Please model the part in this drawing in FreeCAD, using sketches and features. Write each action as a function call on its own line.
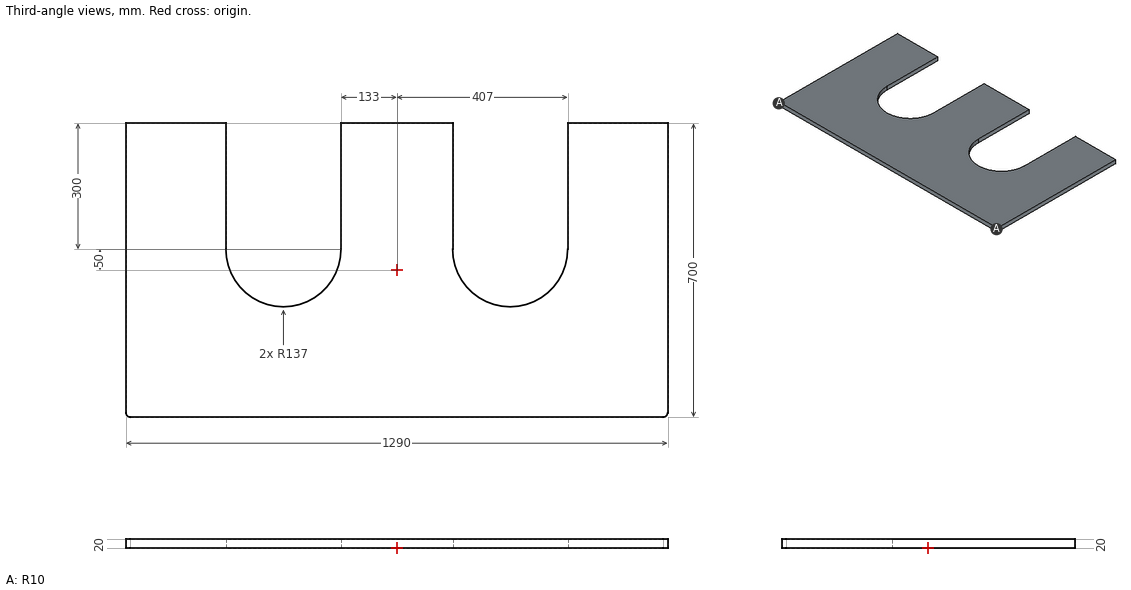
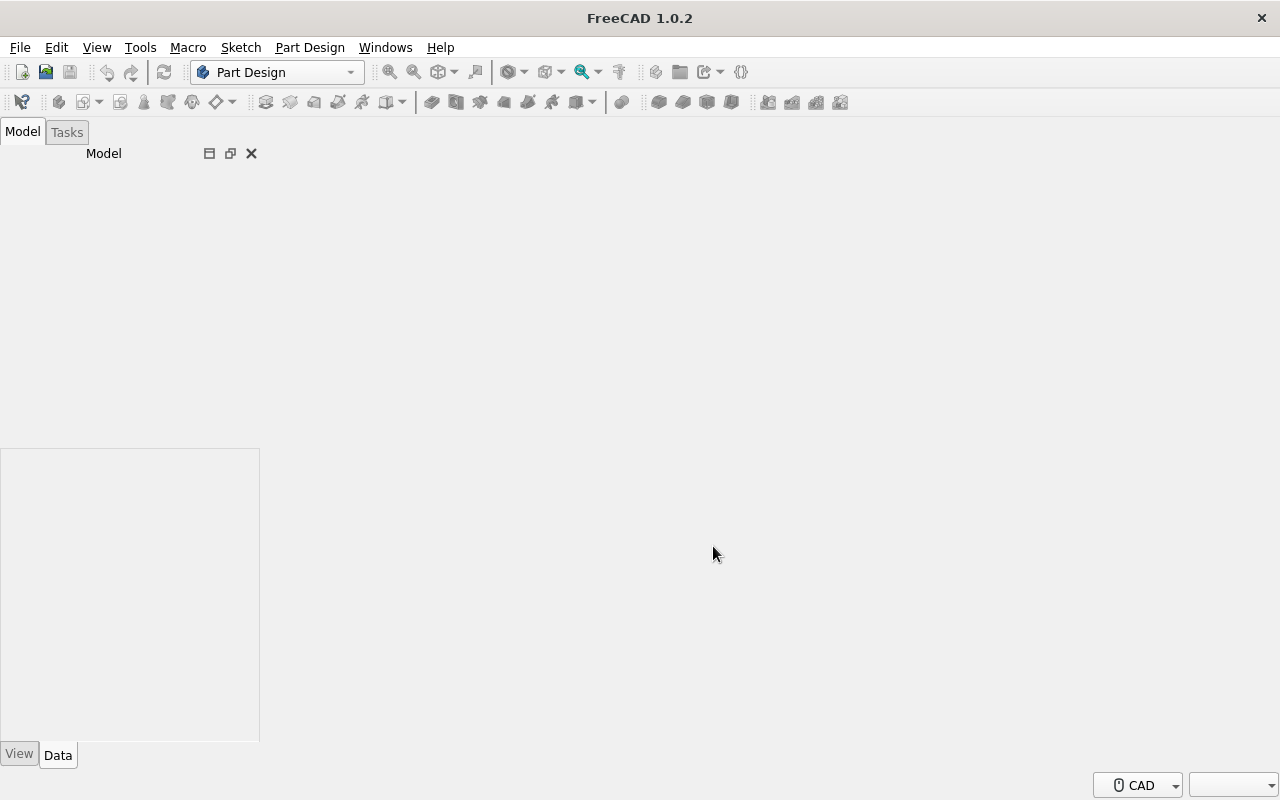
key(ctrl+n)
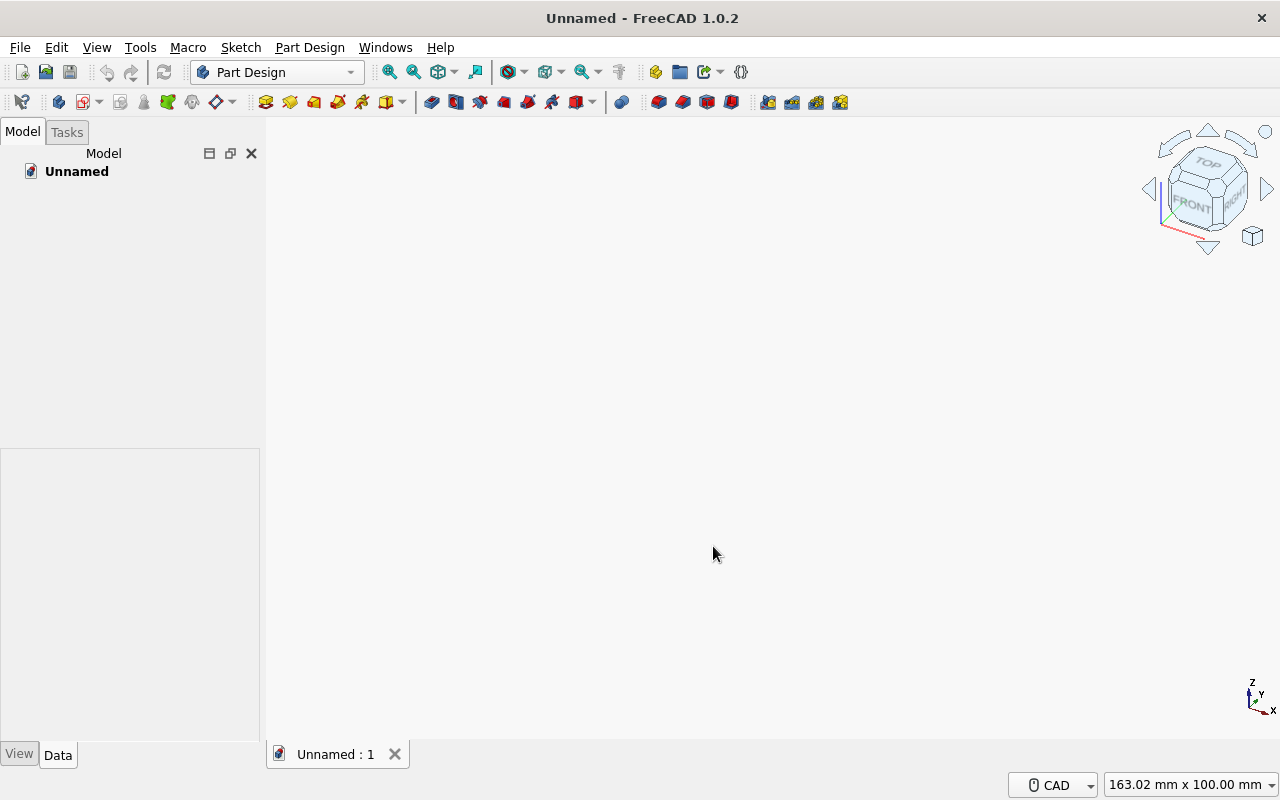
click(84, 102)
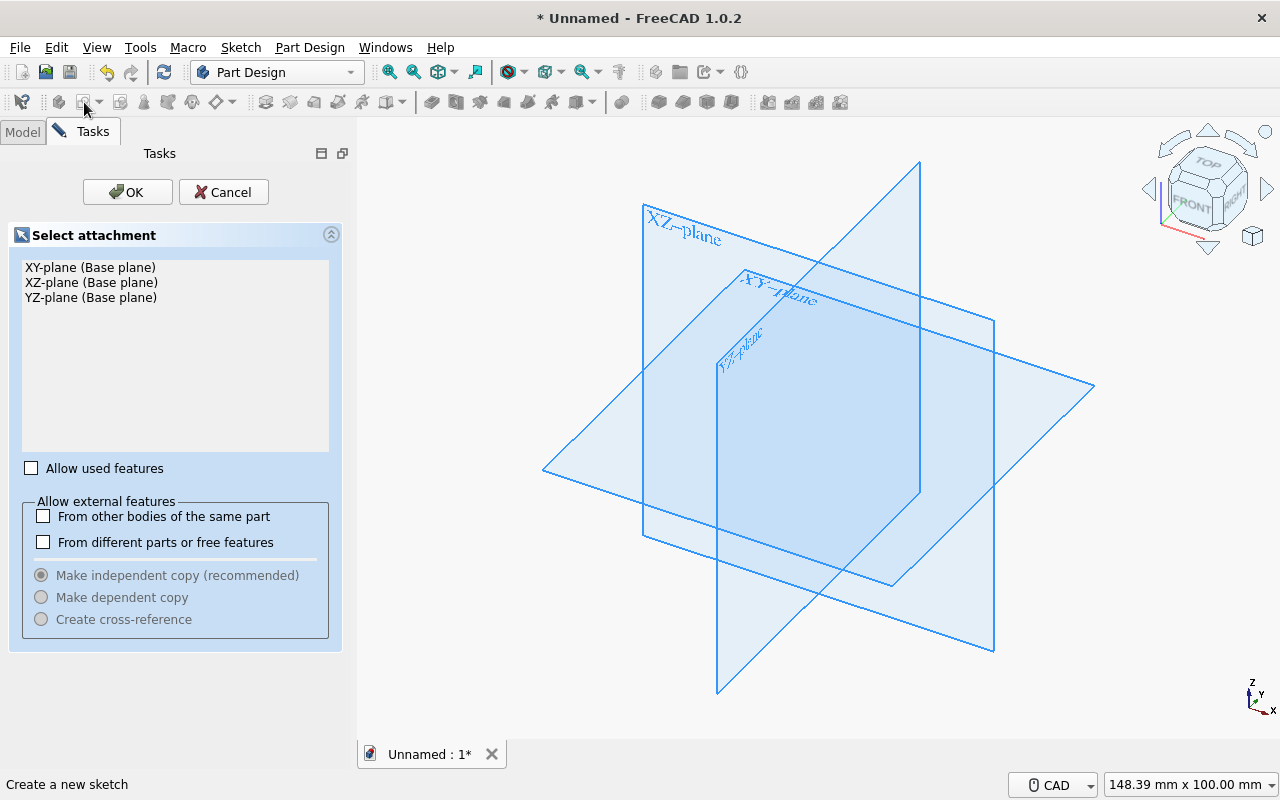
click(82, 268)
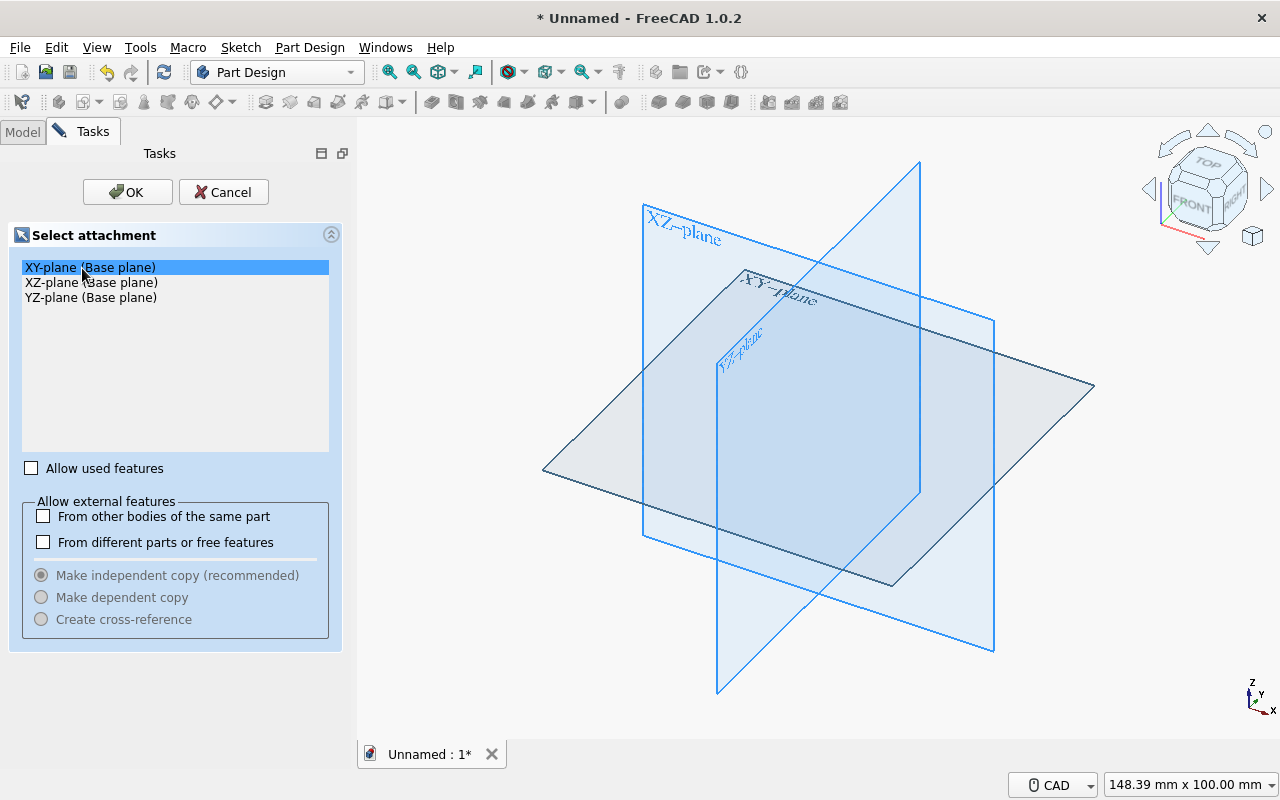
click(128, 192)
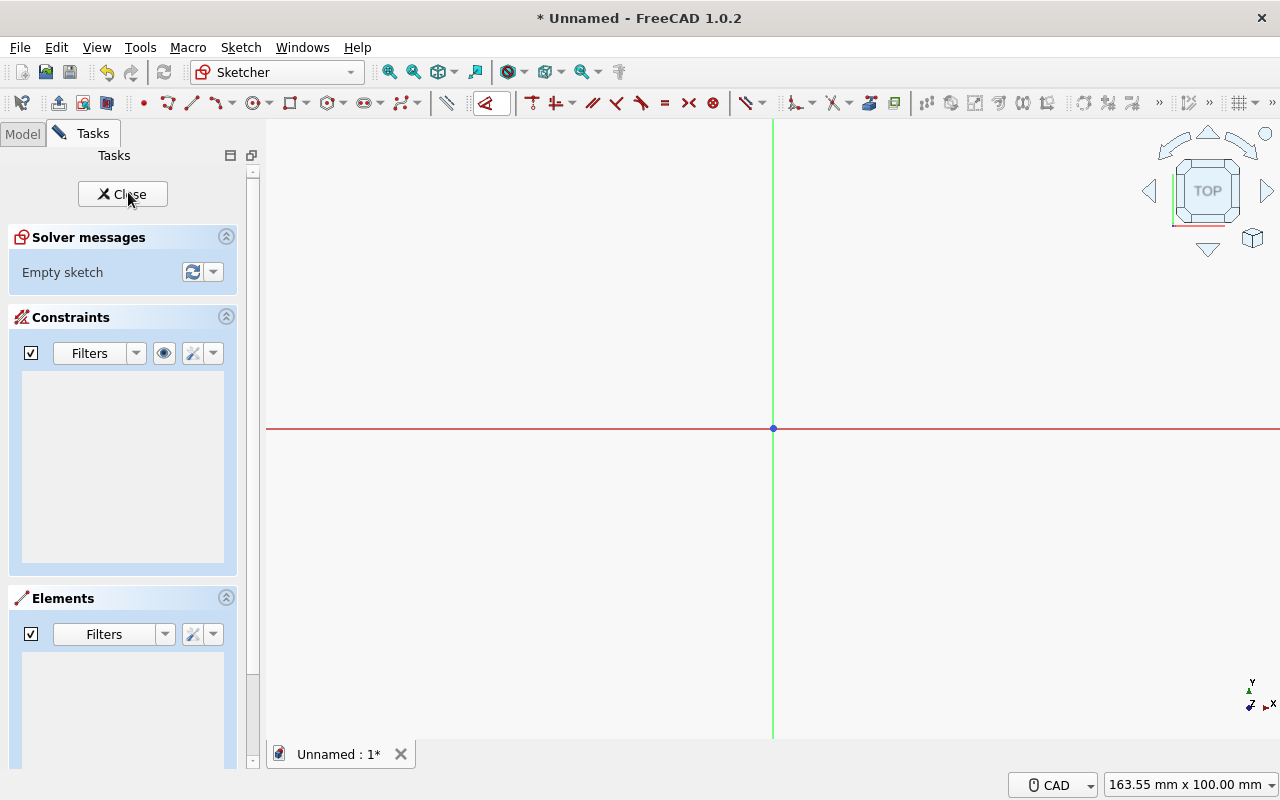
scroll(699, 429, down, 13)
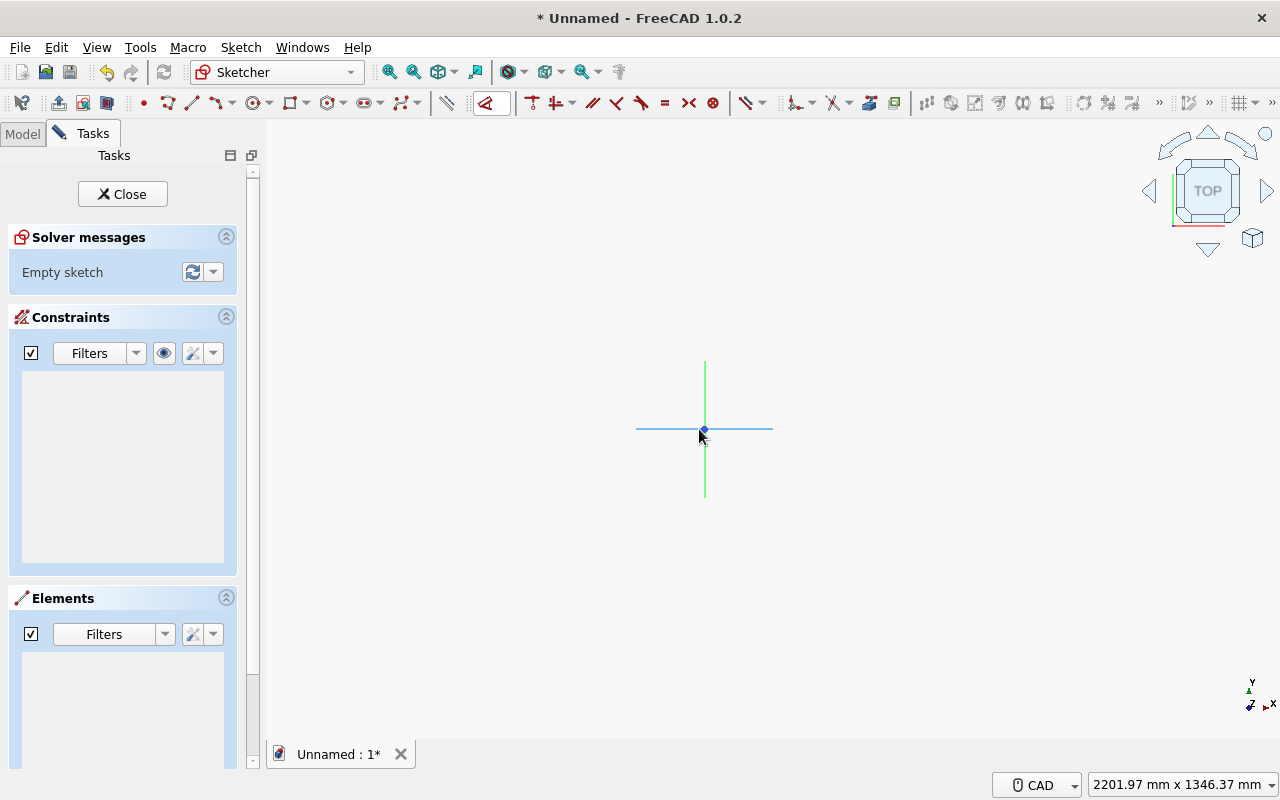
key(g)
key(v)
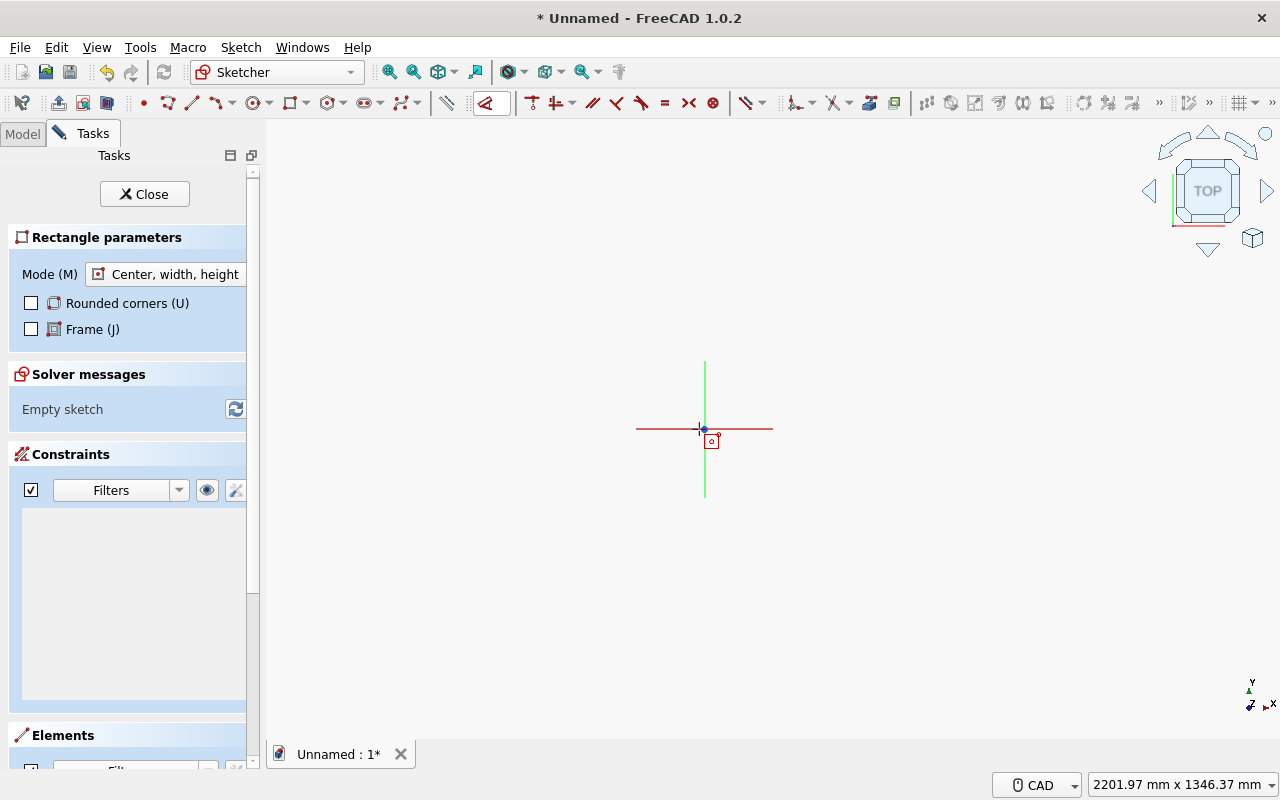
click(705, 429)
move(1002, 268)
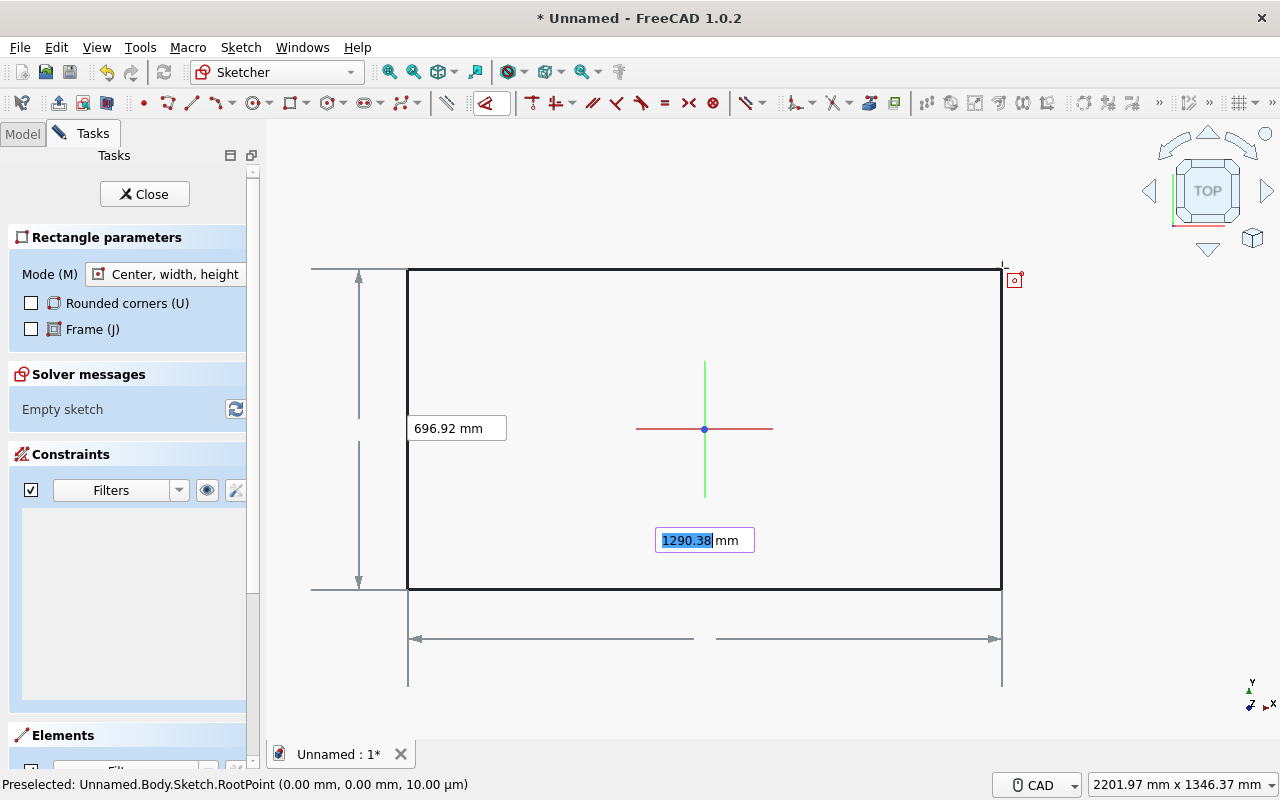
text(1290)
key(Tab)
text(700)
key(Return)
key(Escape)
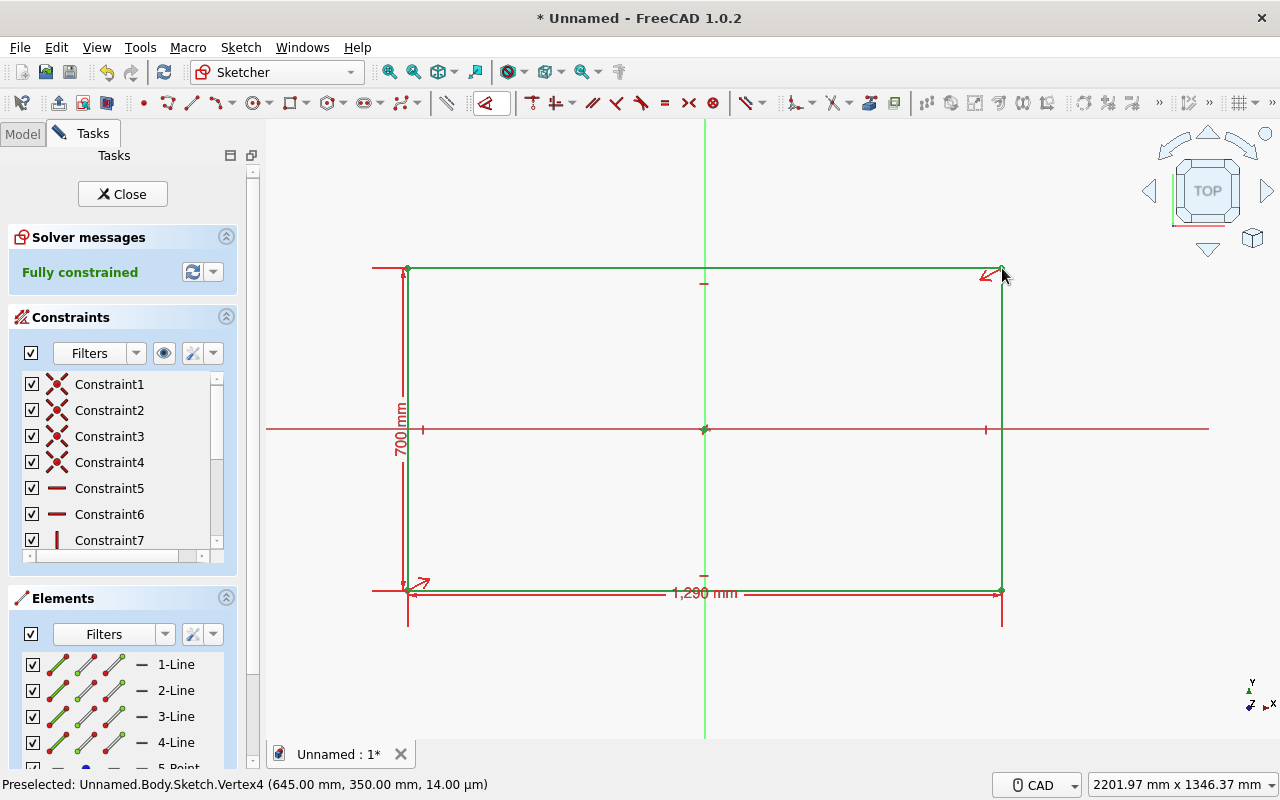
click(123, 194)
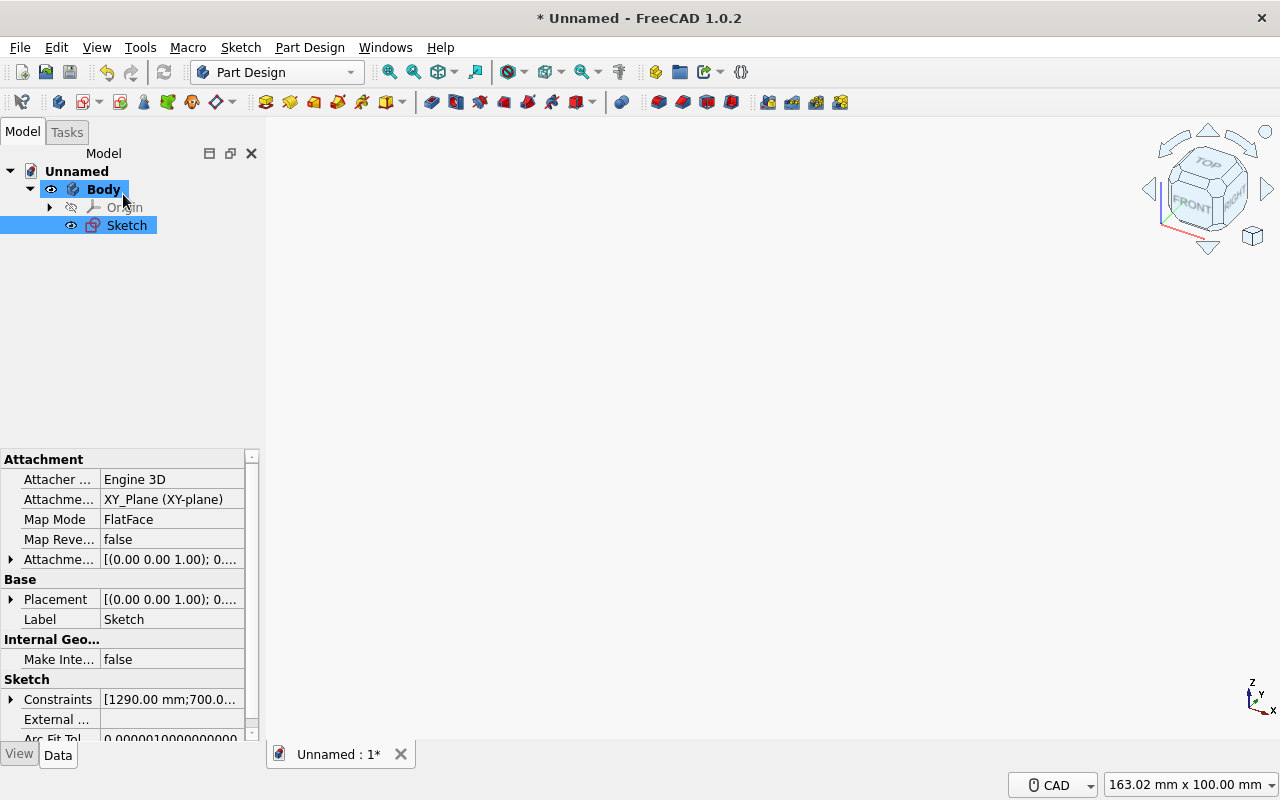
click(266, 102)